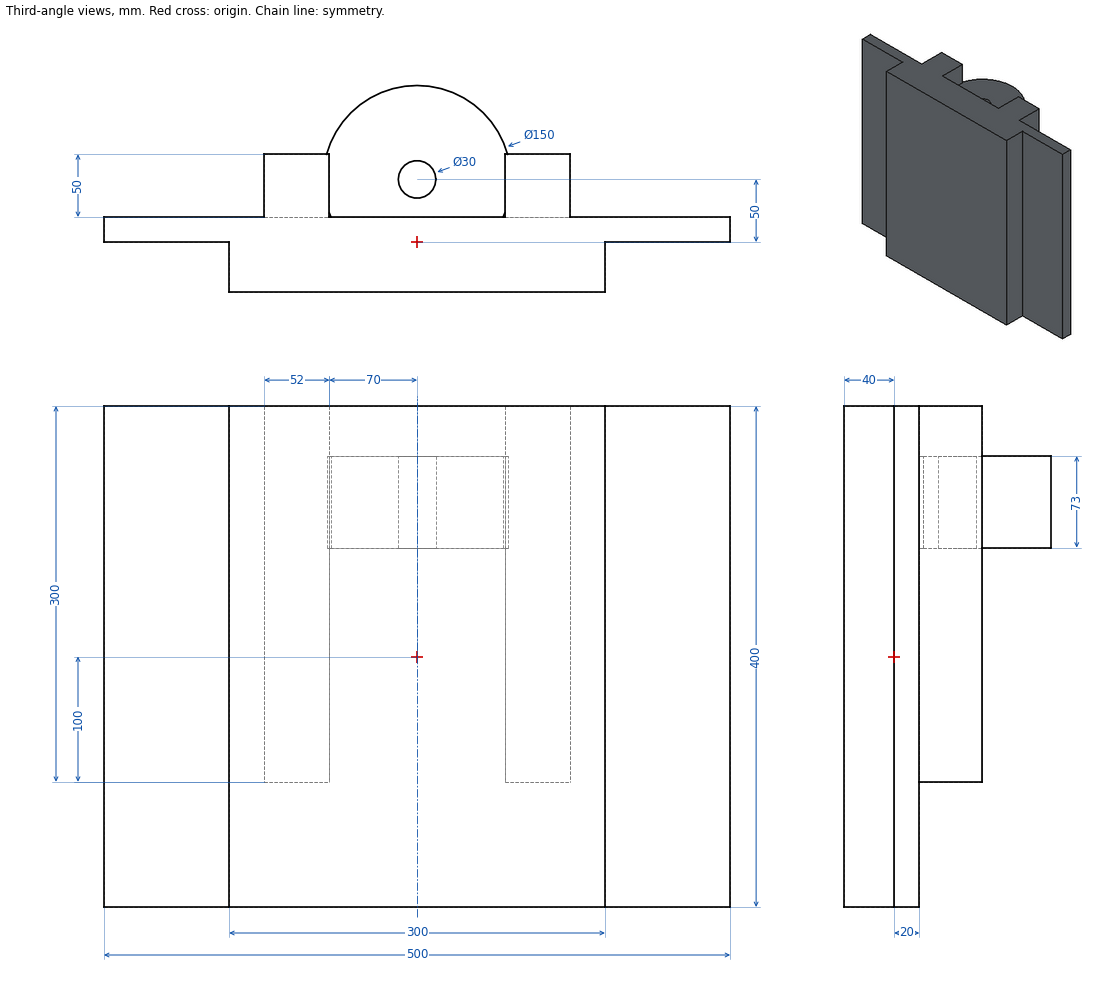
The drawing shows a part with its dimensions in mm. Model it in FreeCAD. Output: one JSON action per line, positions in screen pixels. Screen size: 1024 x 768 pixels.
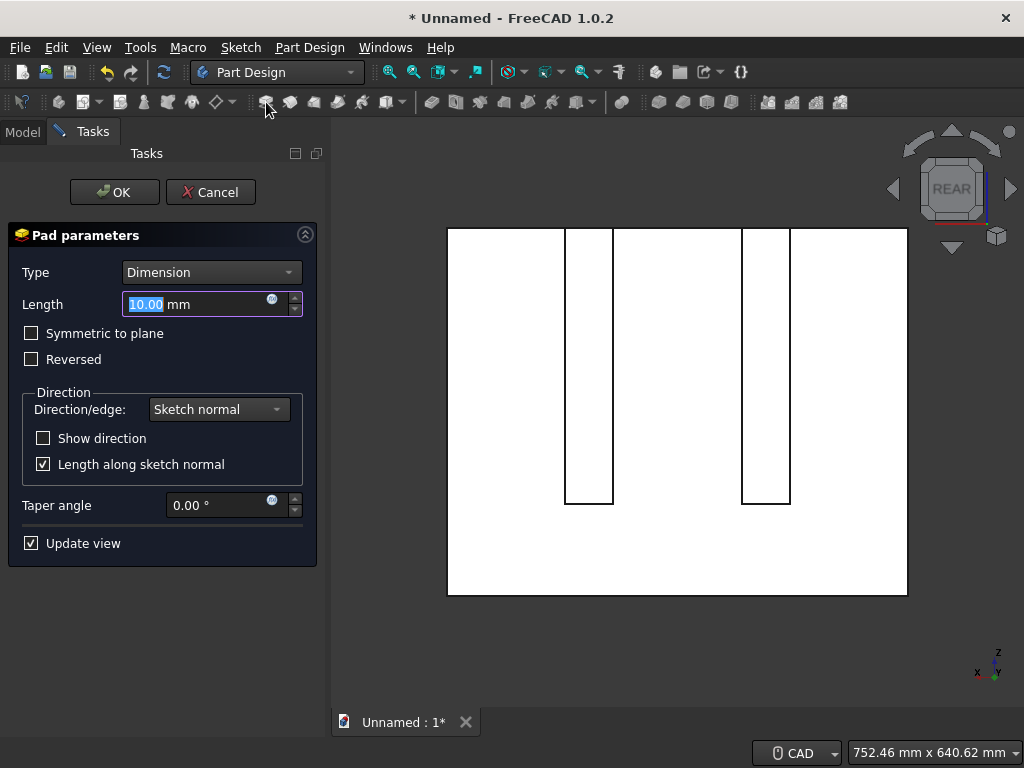
{"action": "type", "text": "40"}
{"action": "key", "text": "Tab"}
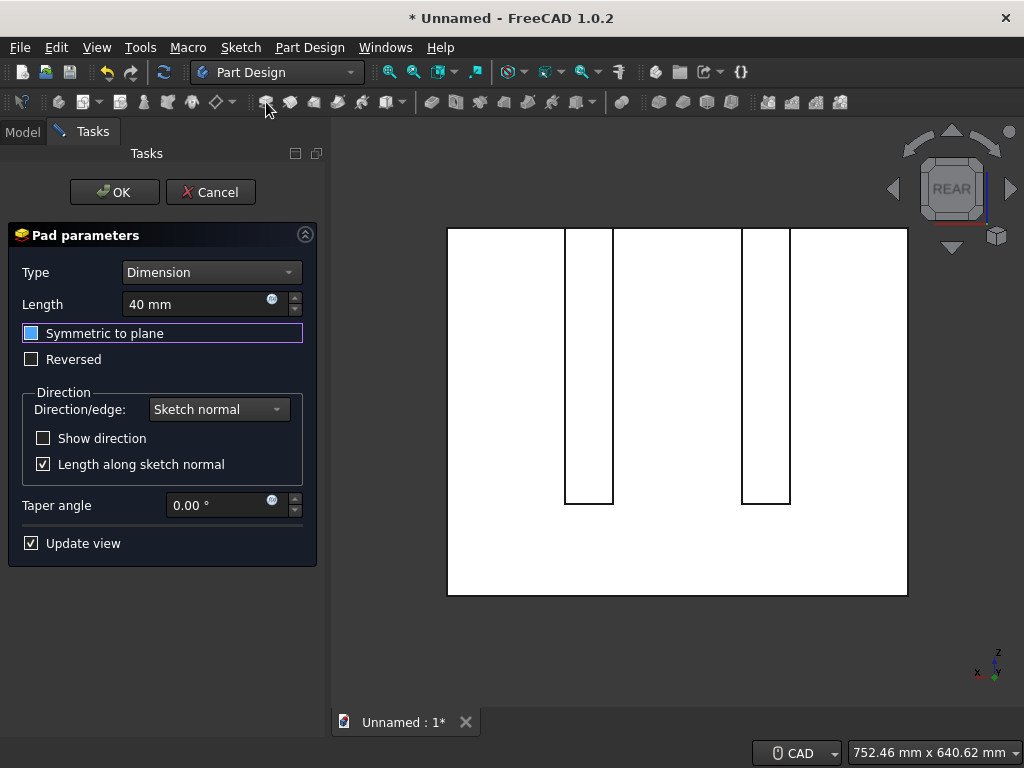
{"action": "left_click", "coordinate": [115, 192]}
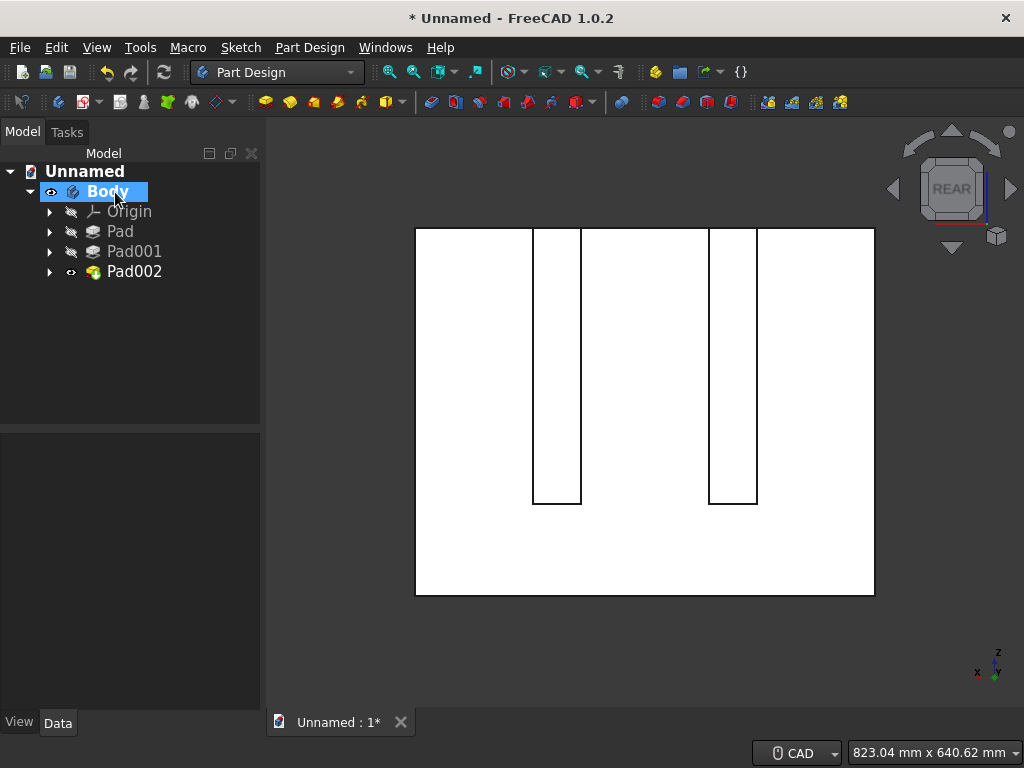
{"action": "left_click", "coordinate": [50, 212]}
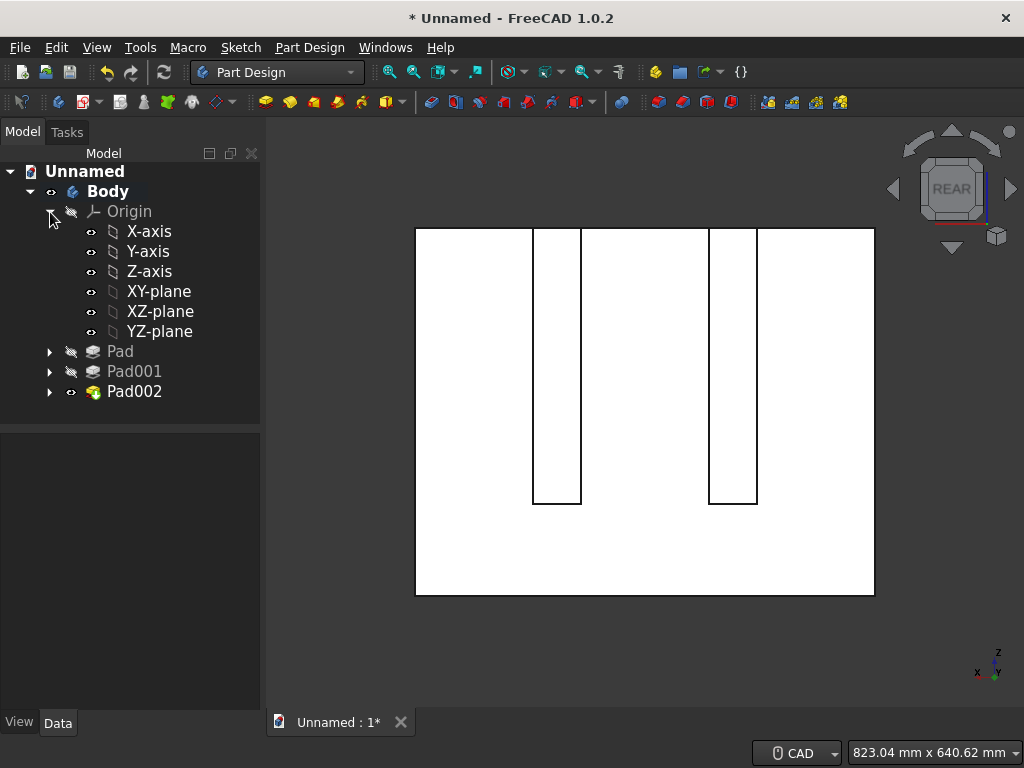
{"action": "left_click", "coordinate": [136, 292]}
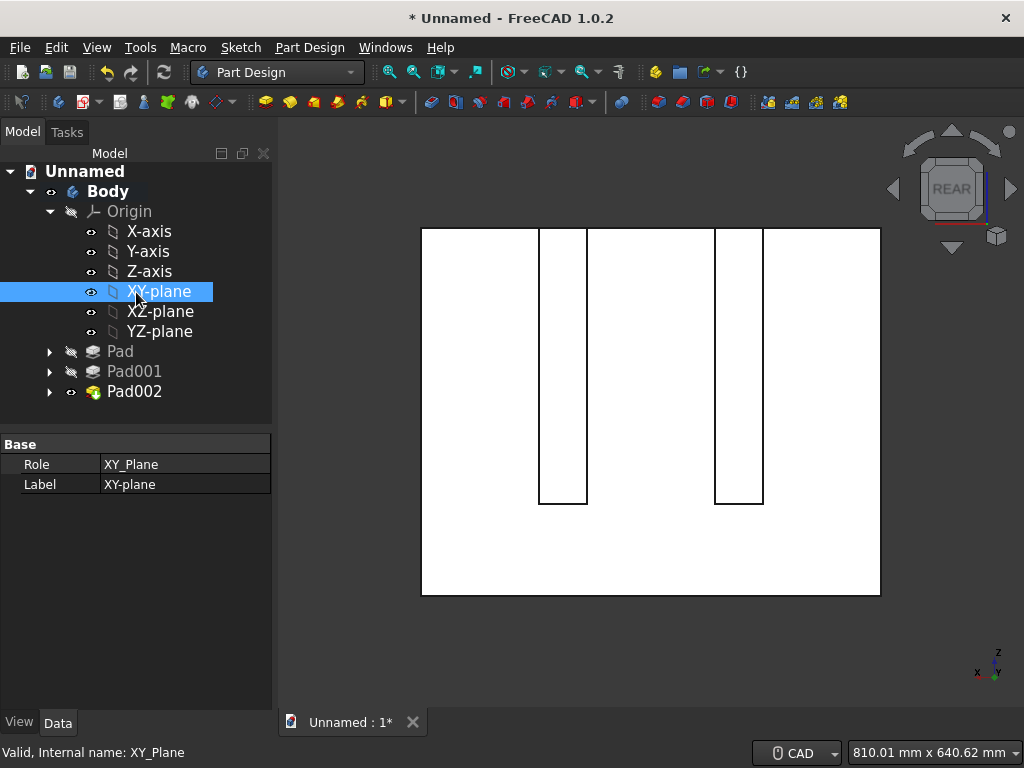
{"action": "left_click", "coordinate": [216, 102]}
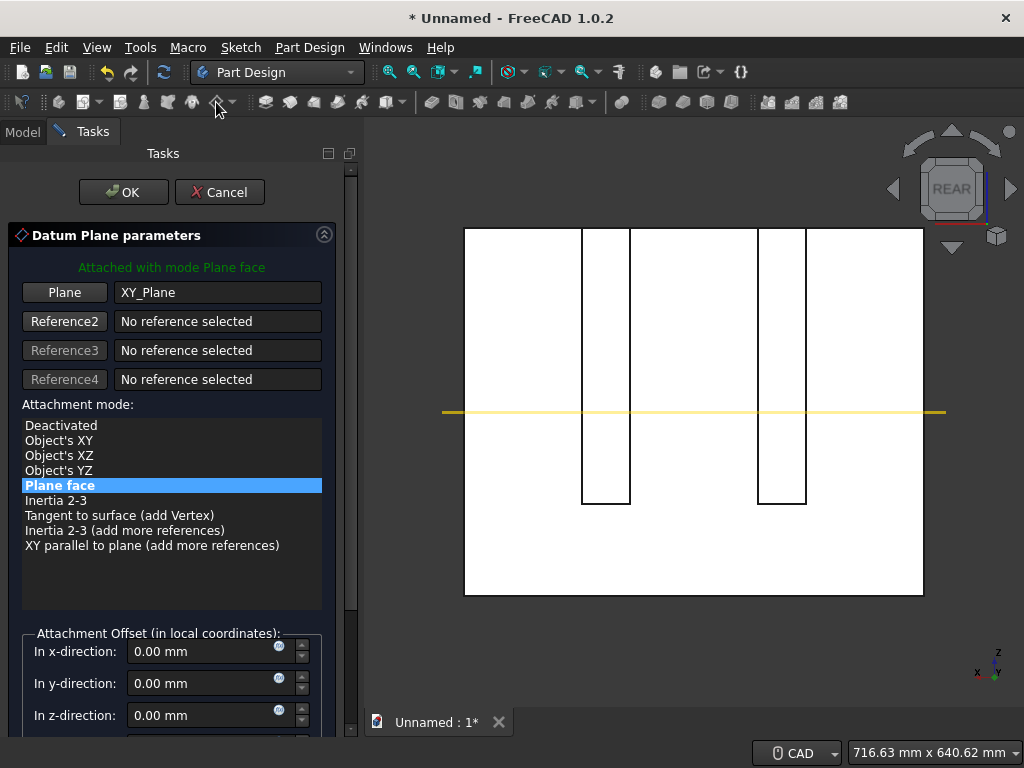
{"action": "triple_click", "coordinate": [210, 715]}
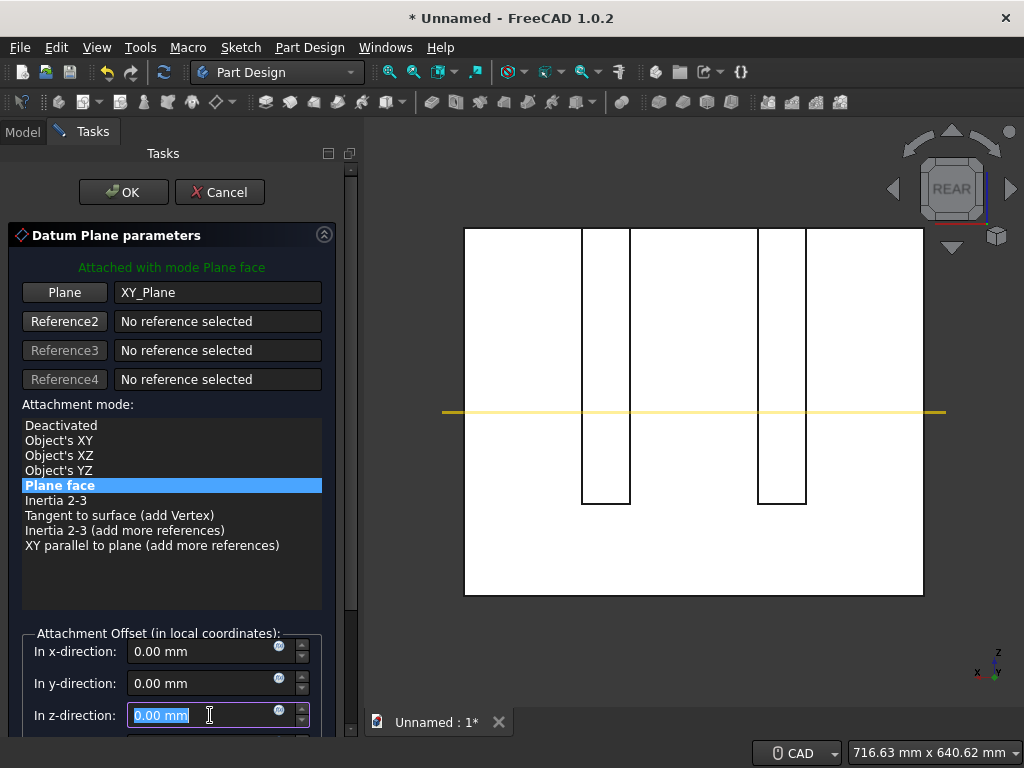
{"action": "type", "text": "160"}
{"action": "key", "text": "Tab"}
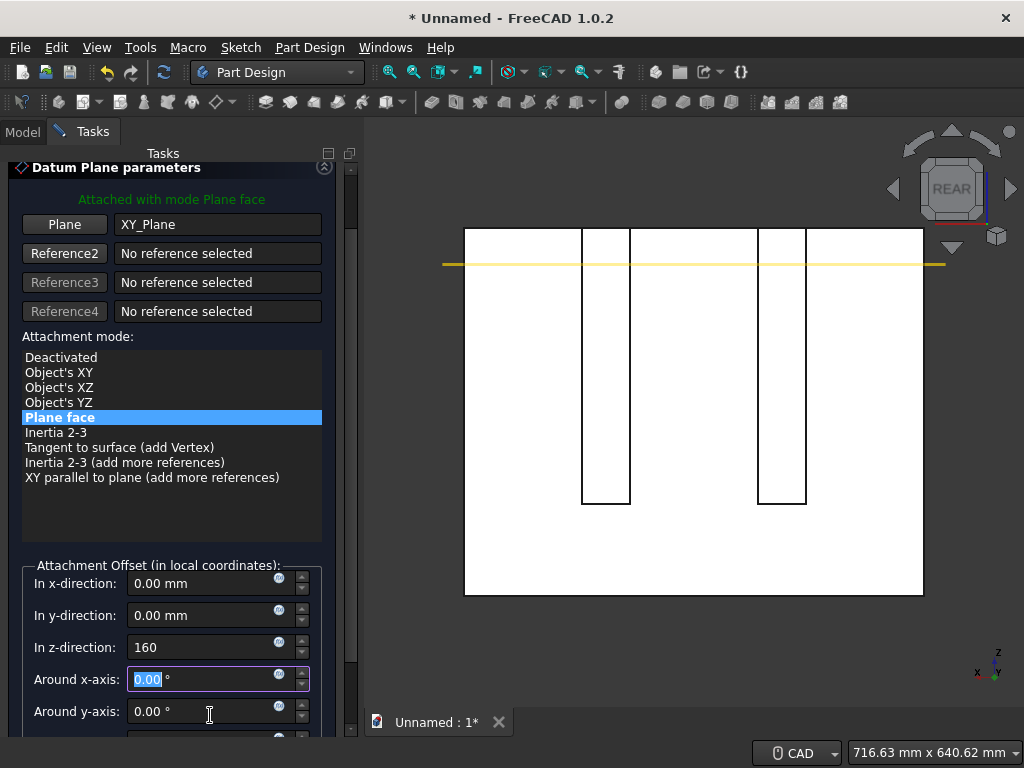
{"action": "scroll", "coordinate": [351, 450], "scroll_direction": "up", "scroll_amount": 2}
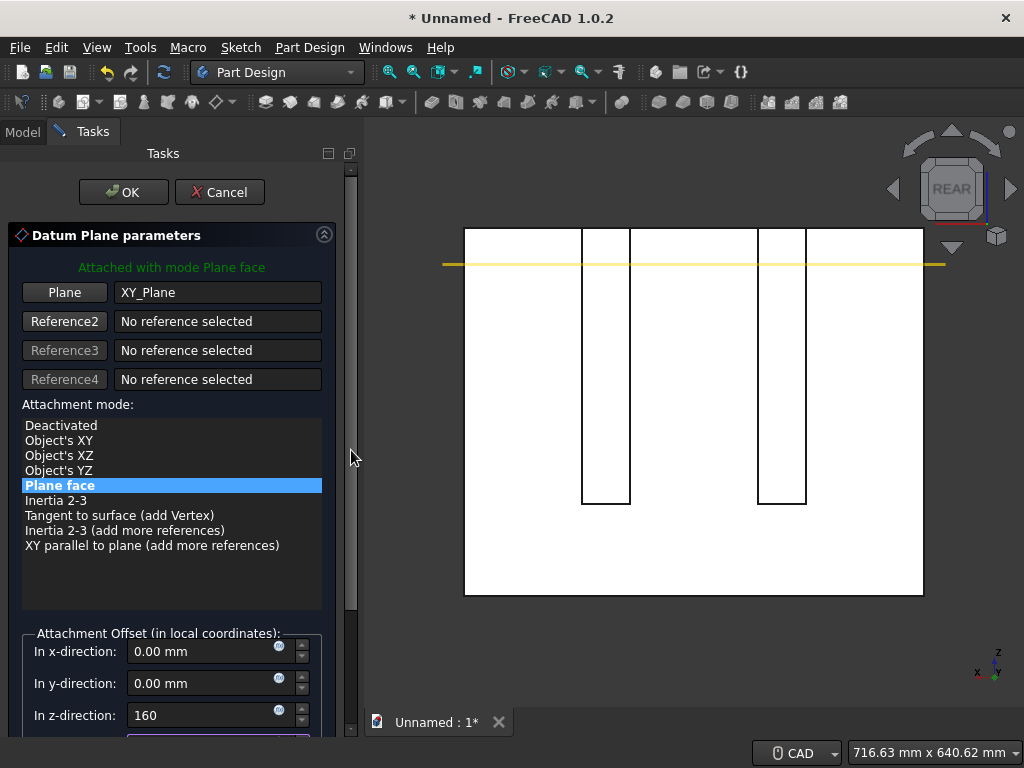
{"action": "left_click", "coordinate": [124, 192]}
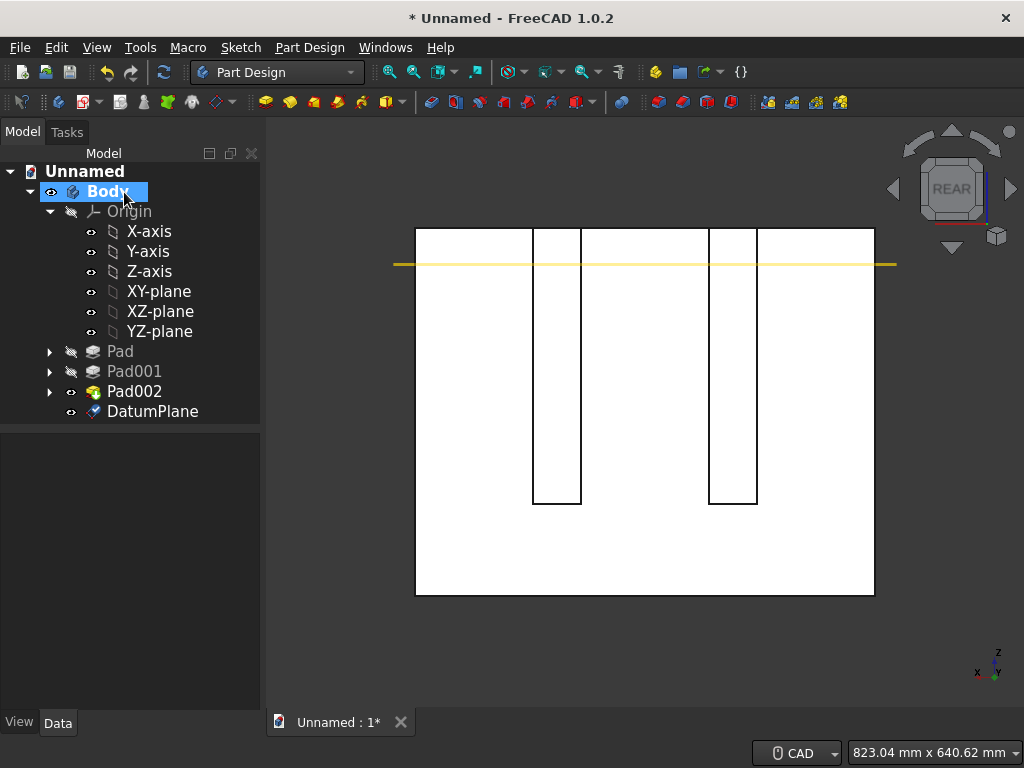
{"action": "left_click", "coordinate": [116, 412]}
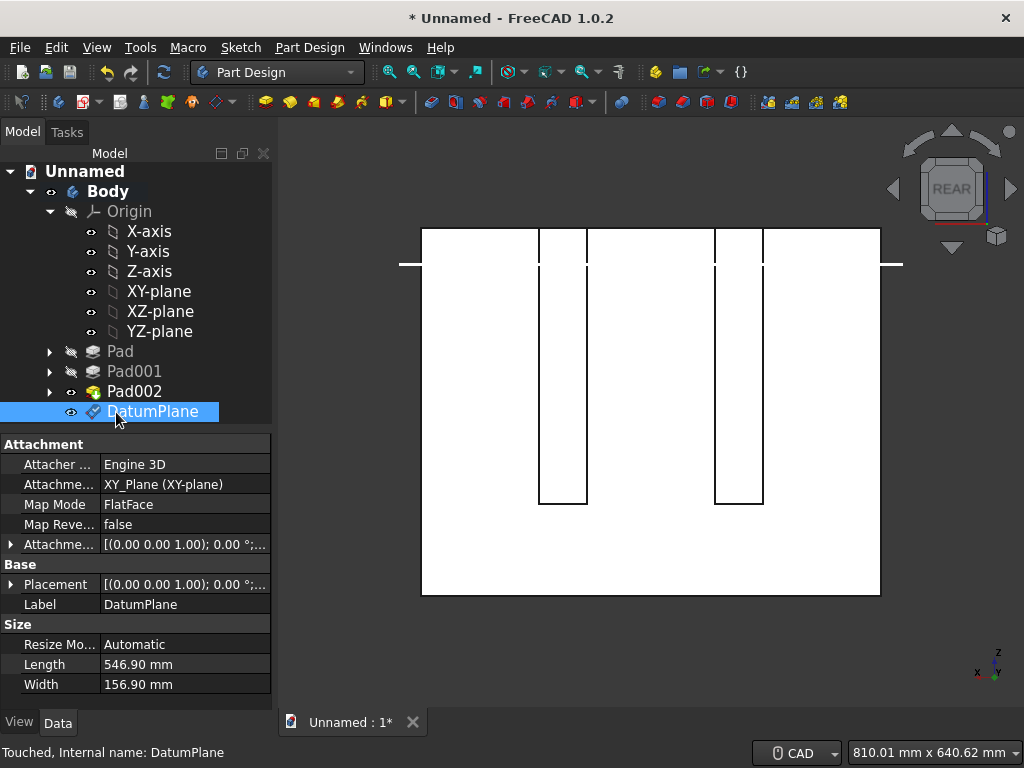
{"action": "left_click", "coordinate": [84, 102]}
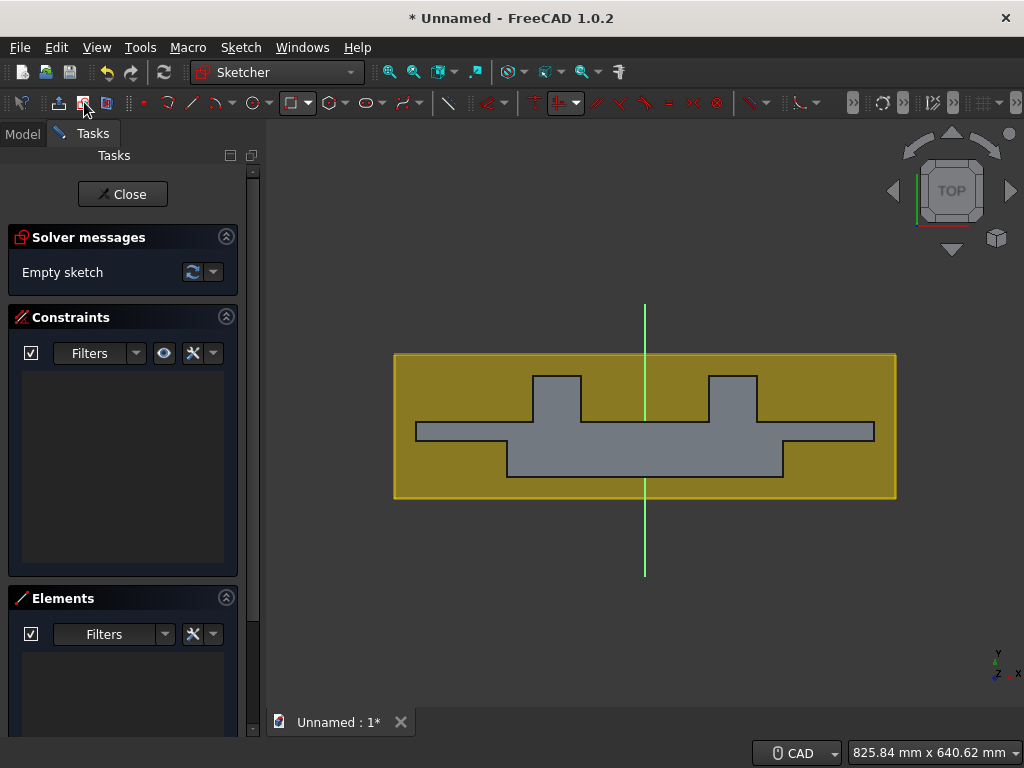
{"action": "left_click", "coordinate": [108, 104]}